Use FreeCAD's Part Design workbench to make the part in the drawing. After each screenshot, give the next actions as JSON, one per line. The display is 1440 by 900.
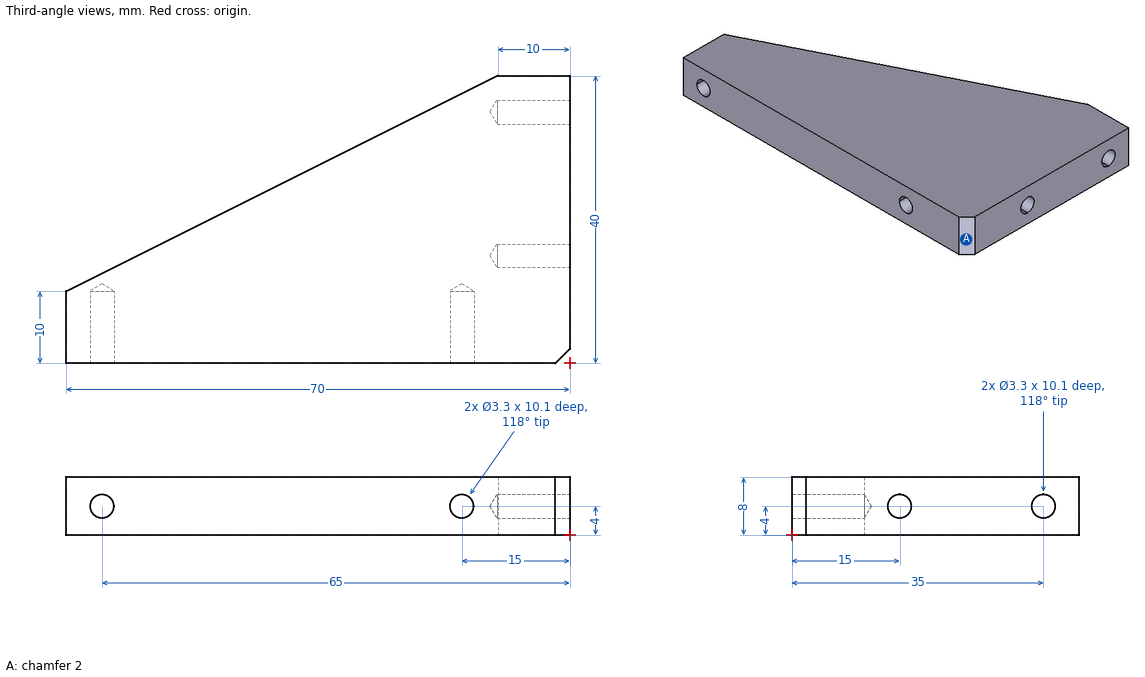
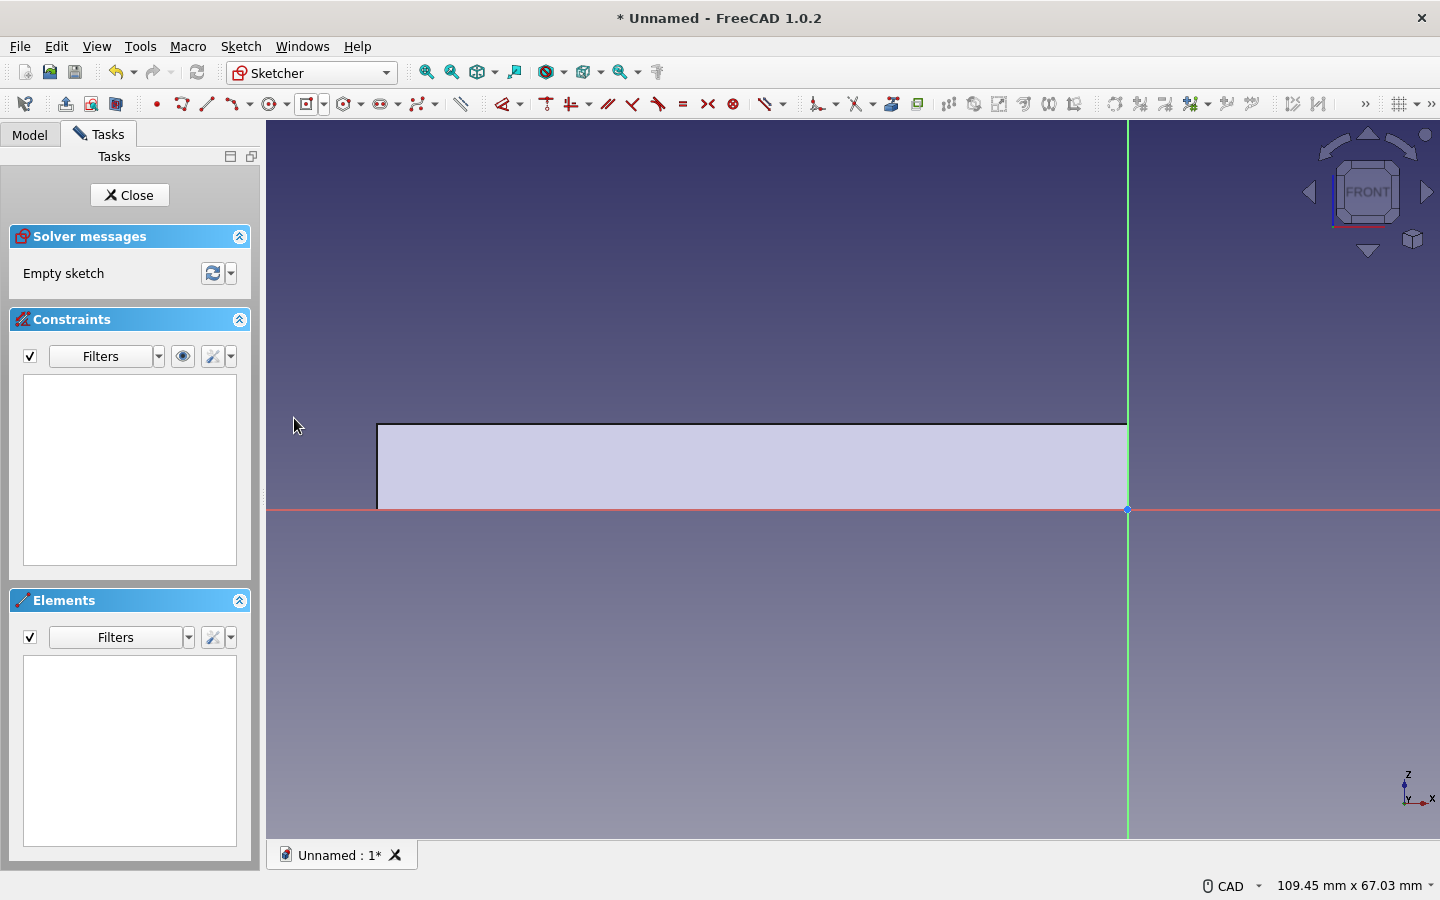
{"action": "left_click", "coordinate": [268, 104]}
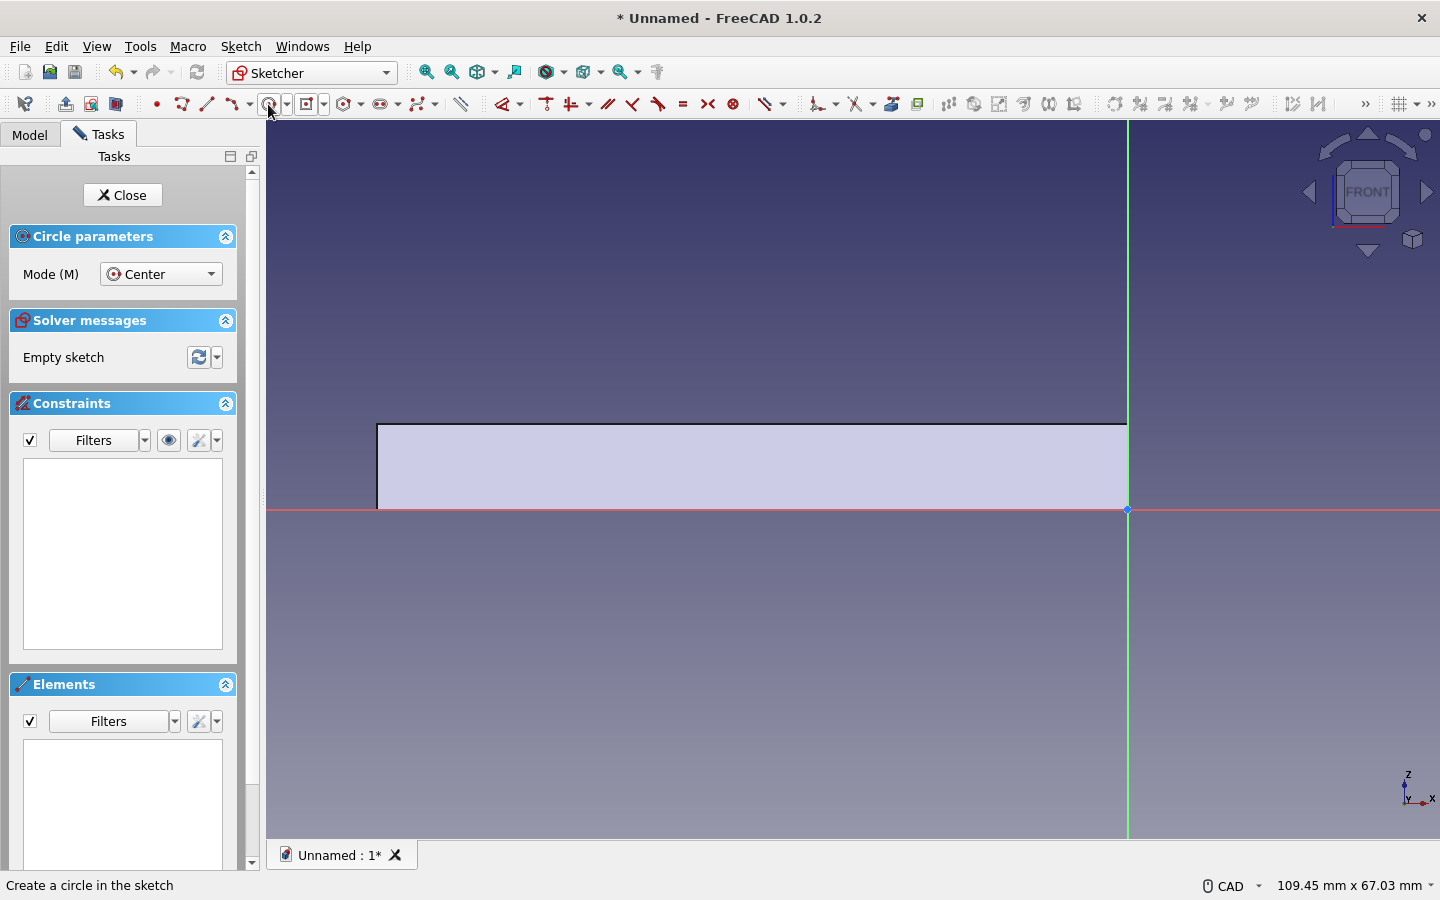
{"action": "scroll", "coordinate": [967, 467], "scroll_direction": "up", "scroll_amount": 2}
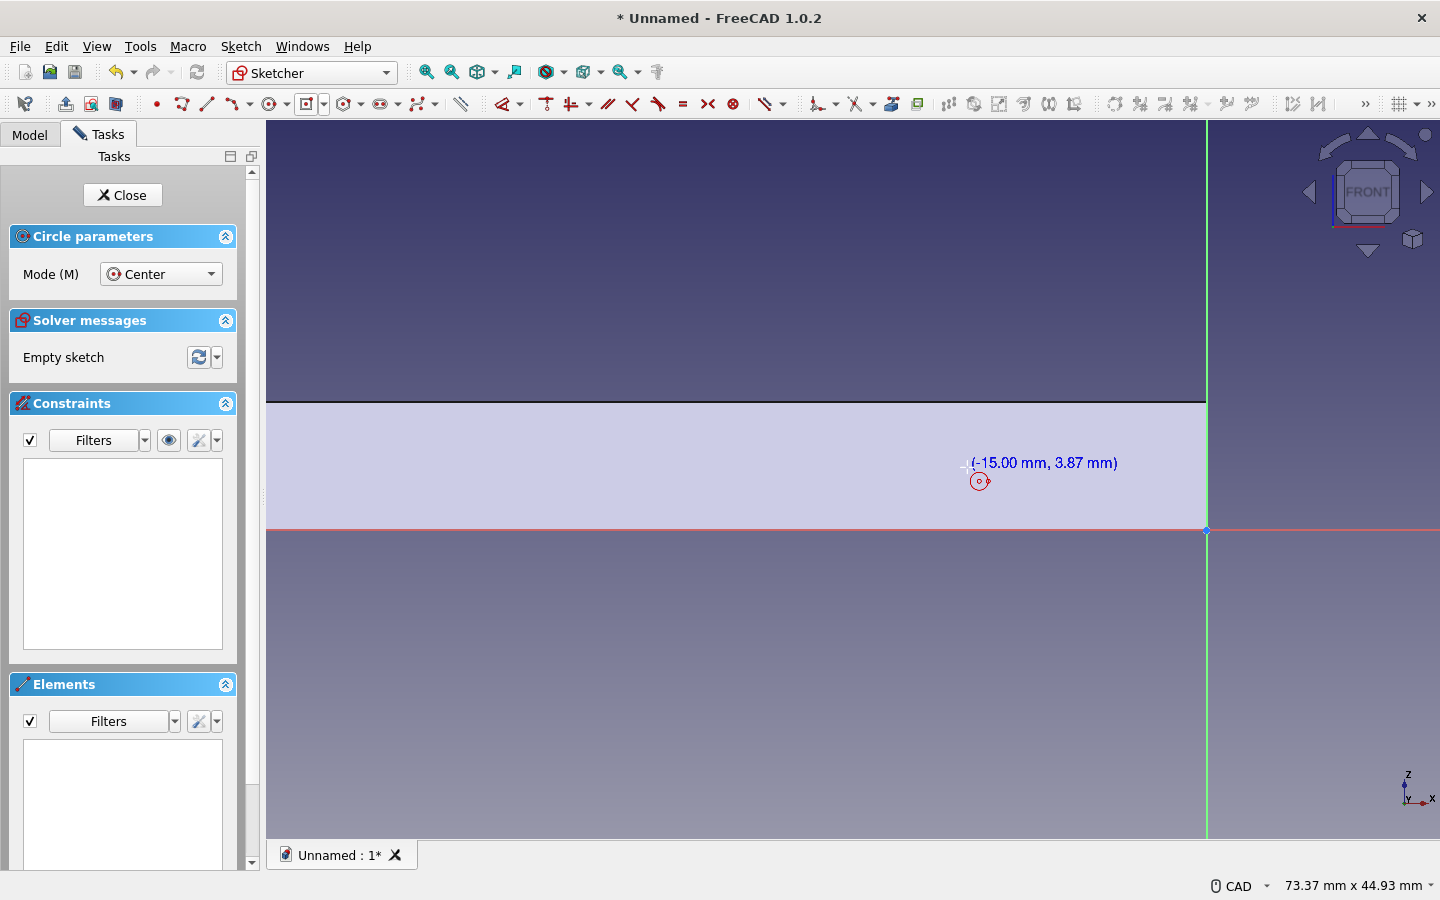
{"action": "left_click", "coordinate": [967, 466]}
{"action": "left_click", "coordinate": [985, 448]}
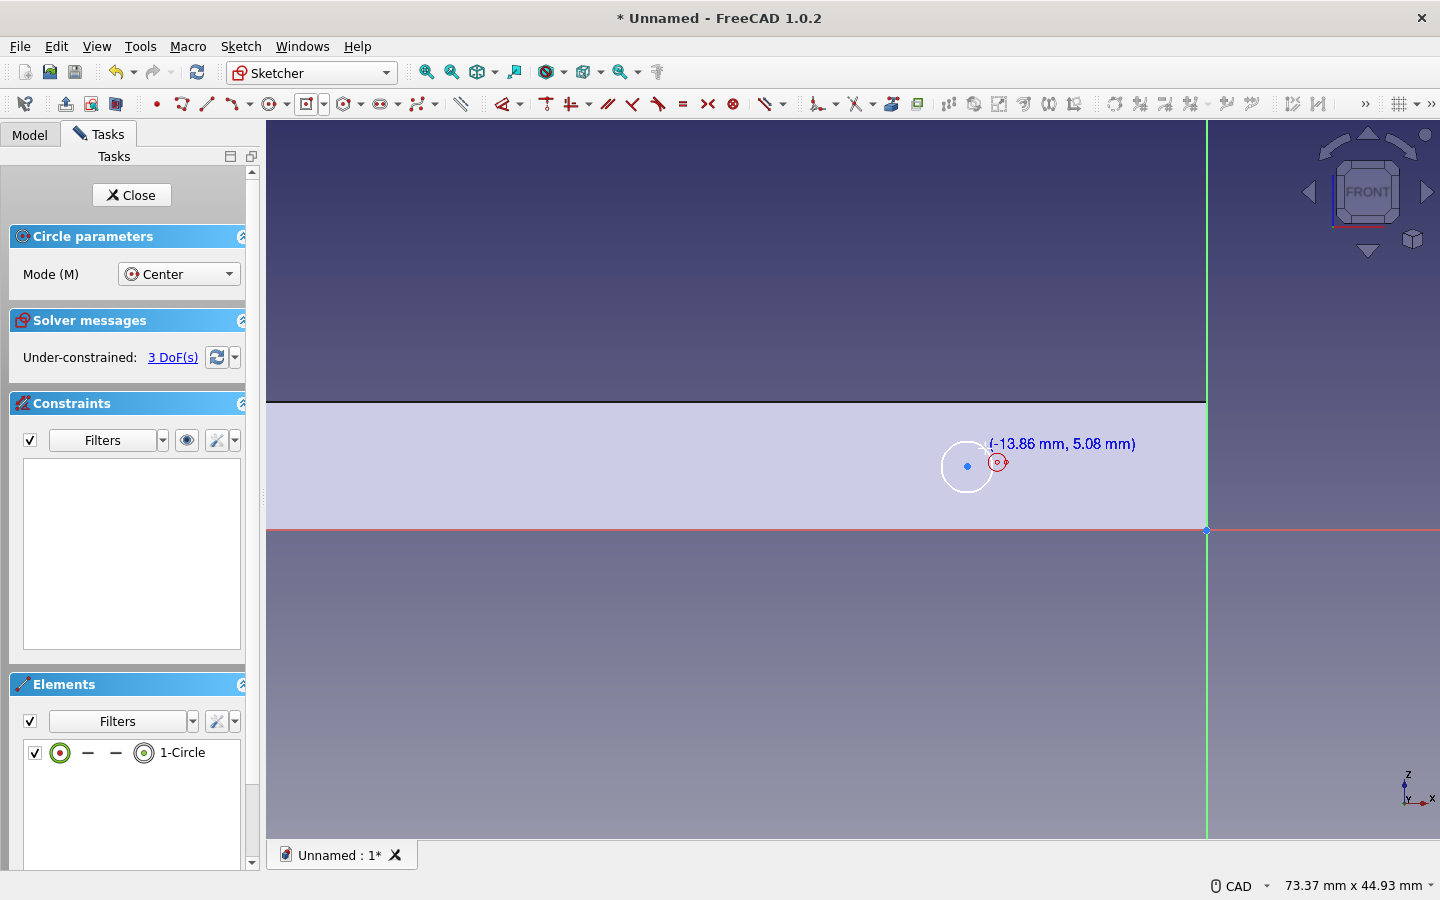
{"action": "scroll", "coordinate": [1010, 468], "scroll_direction": "down", "scroll_amount": 2}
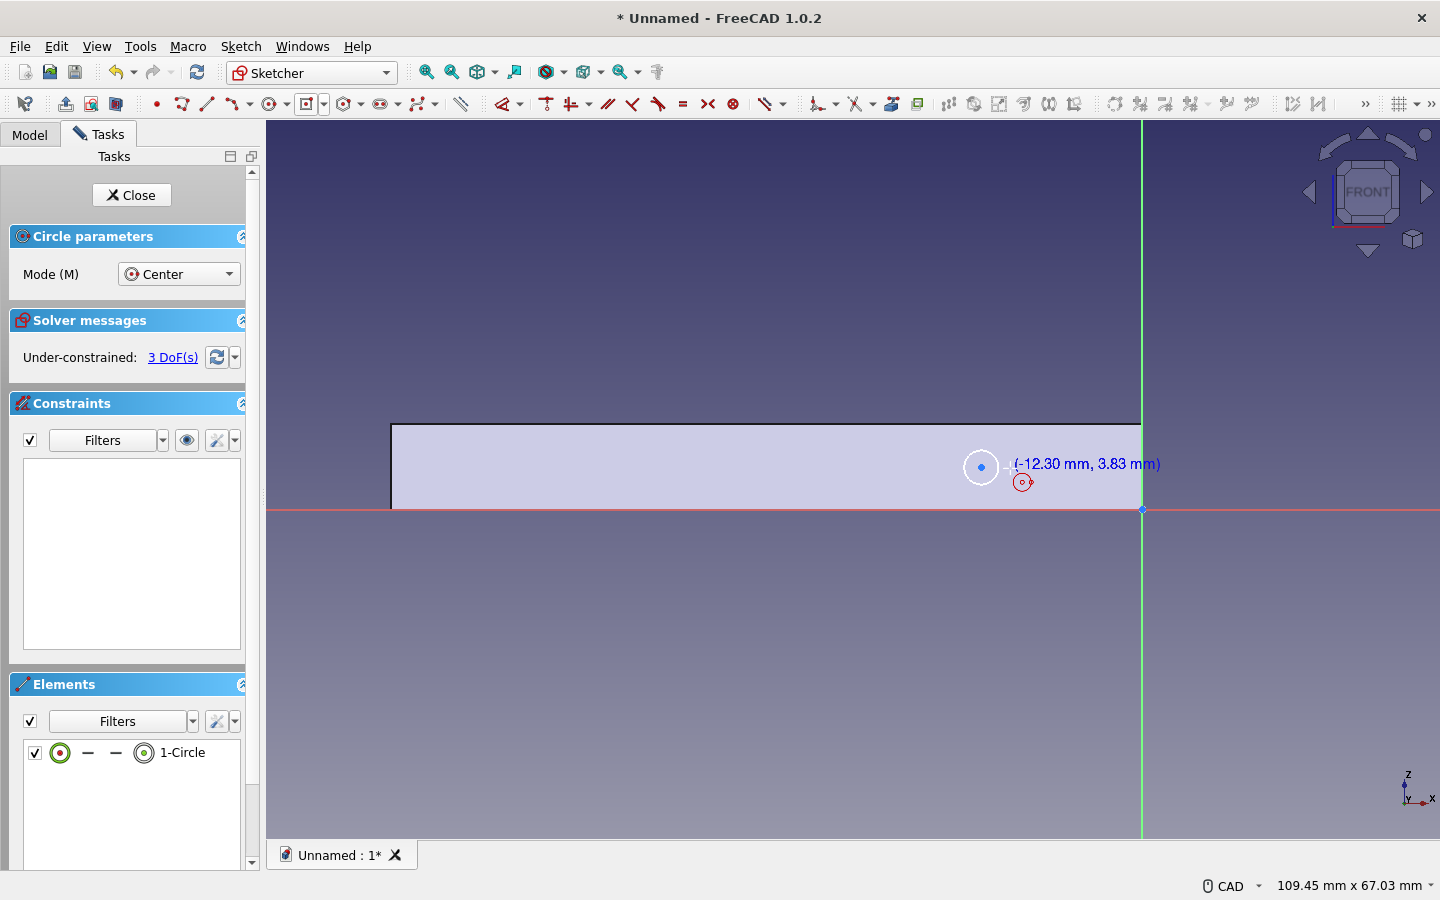
{"action": "scroll", "coordinate": [445, 467], "scroll_direction": "up", "scroll_amount": 2}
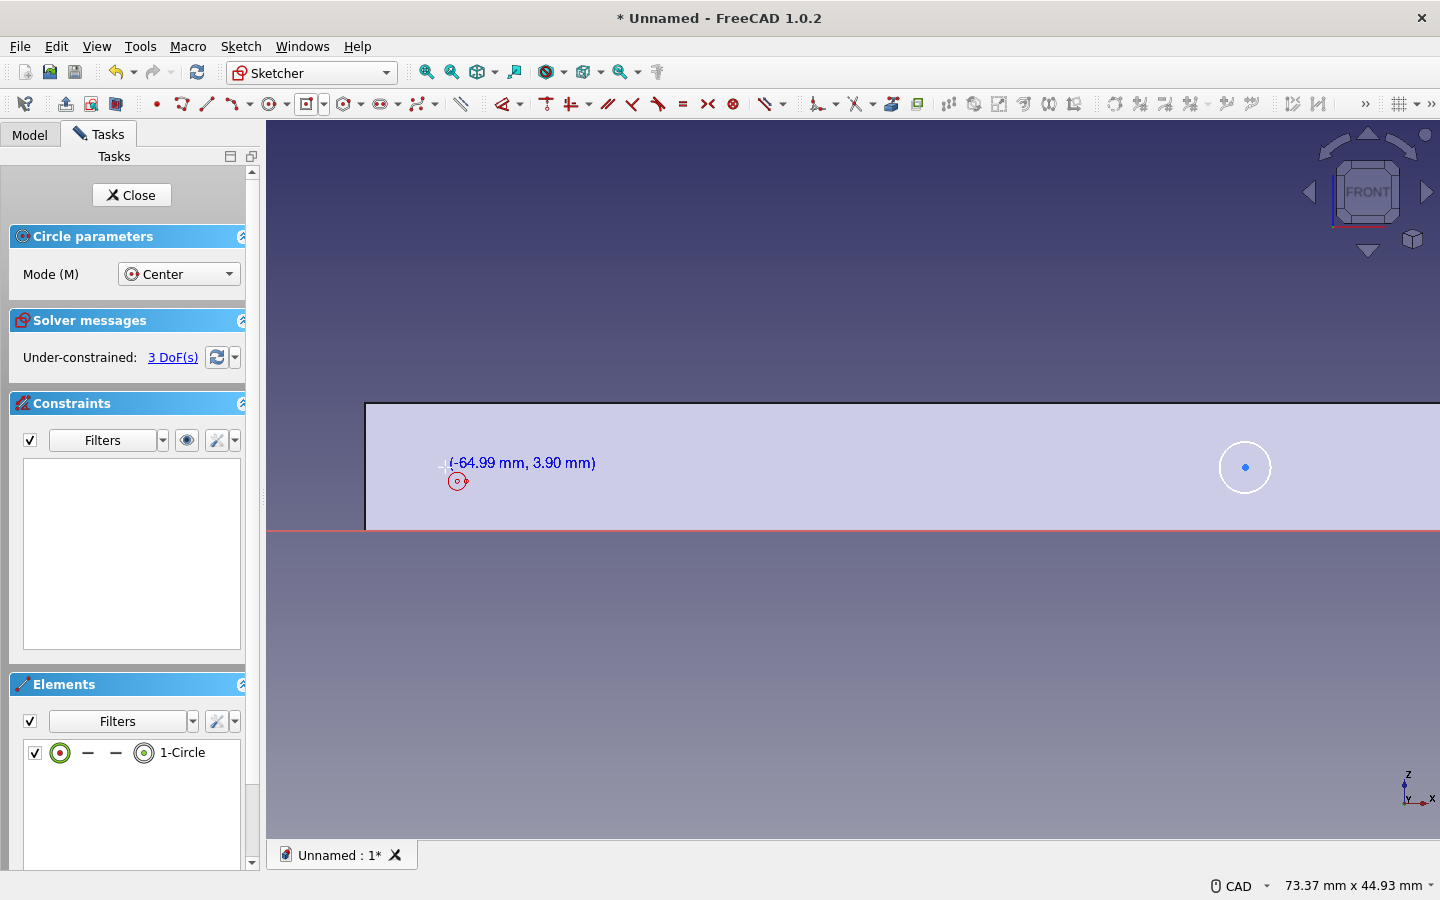
{"action": "left_click", "coordinate": [445, 467]}
{"action": "left_click", "coordinate": [463, 448]}
{"action": "key", "text": "Escape"}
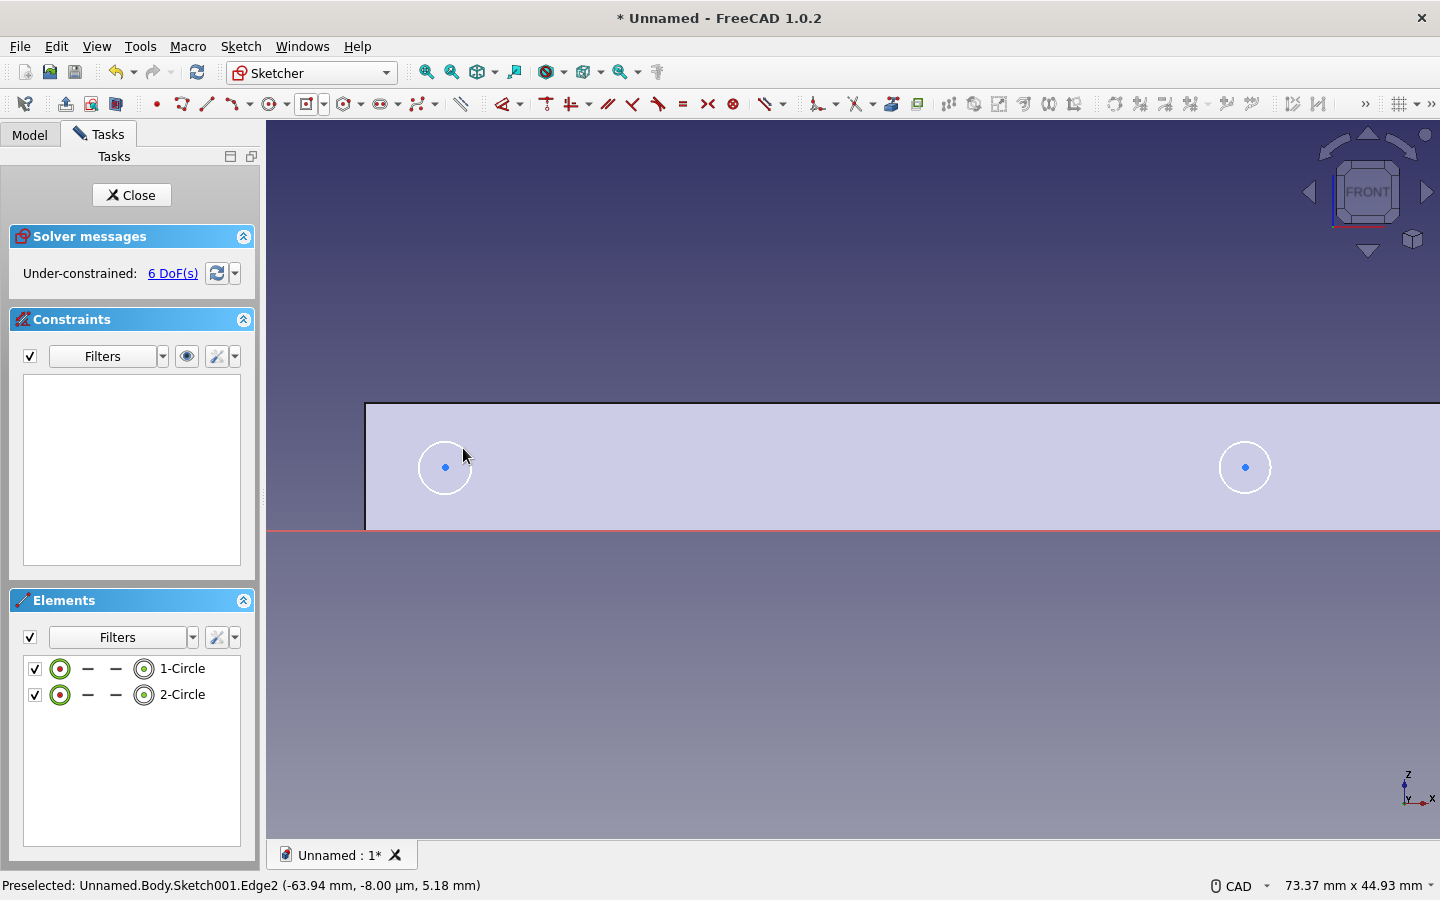
{"action": "left_click", "coordinate": [1263, 449]}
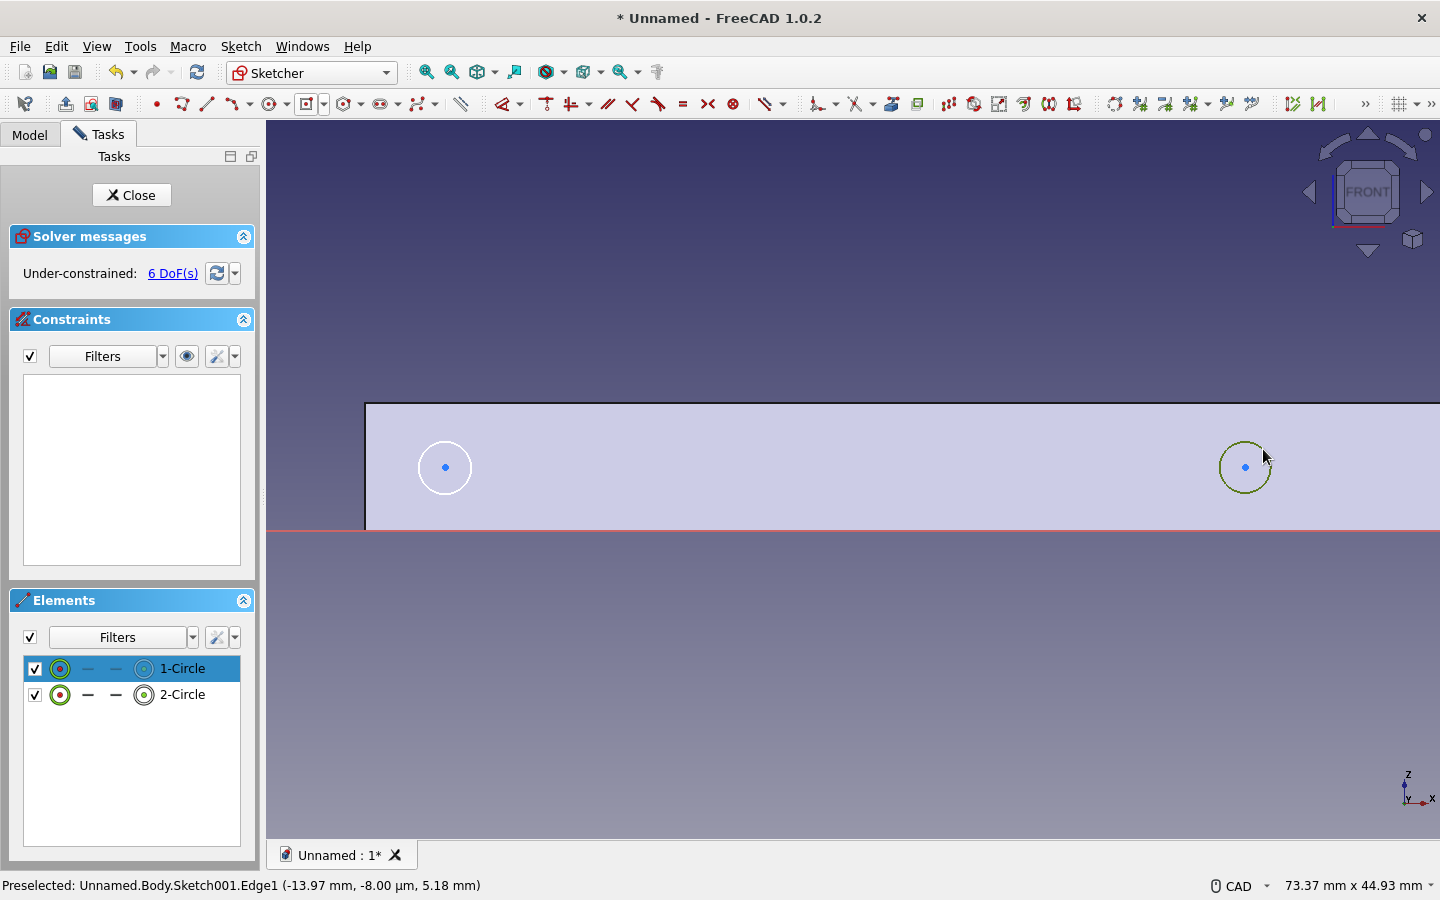
{"action": "left_click", "coordinate": [463, 449]}